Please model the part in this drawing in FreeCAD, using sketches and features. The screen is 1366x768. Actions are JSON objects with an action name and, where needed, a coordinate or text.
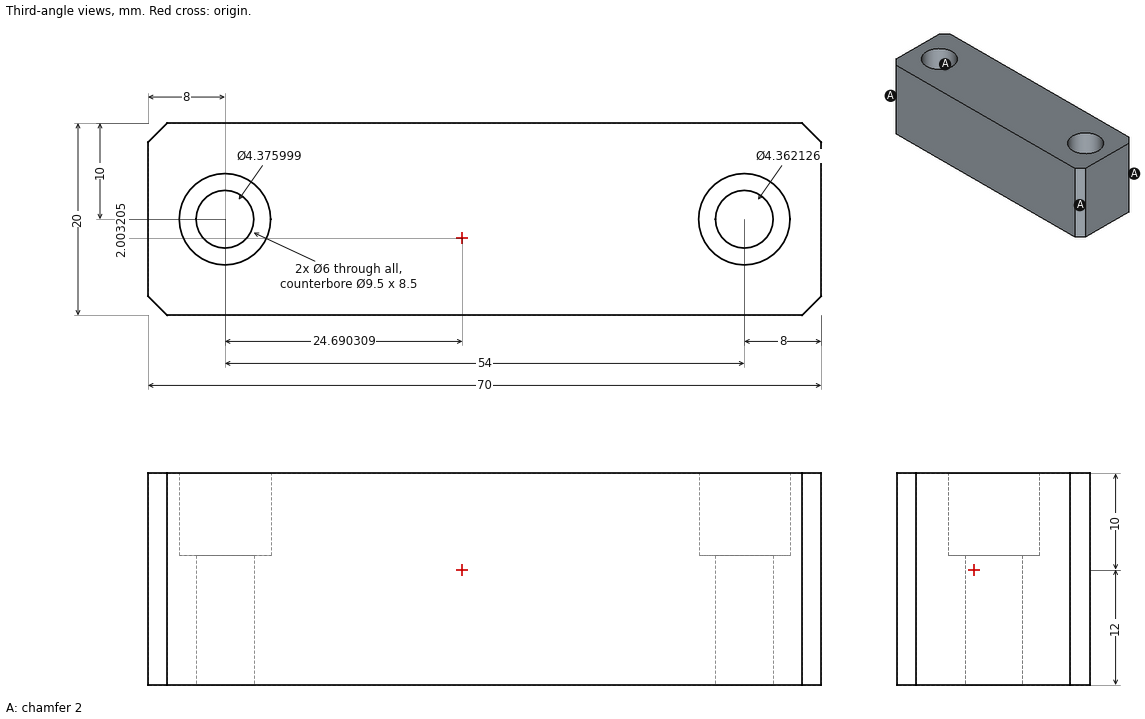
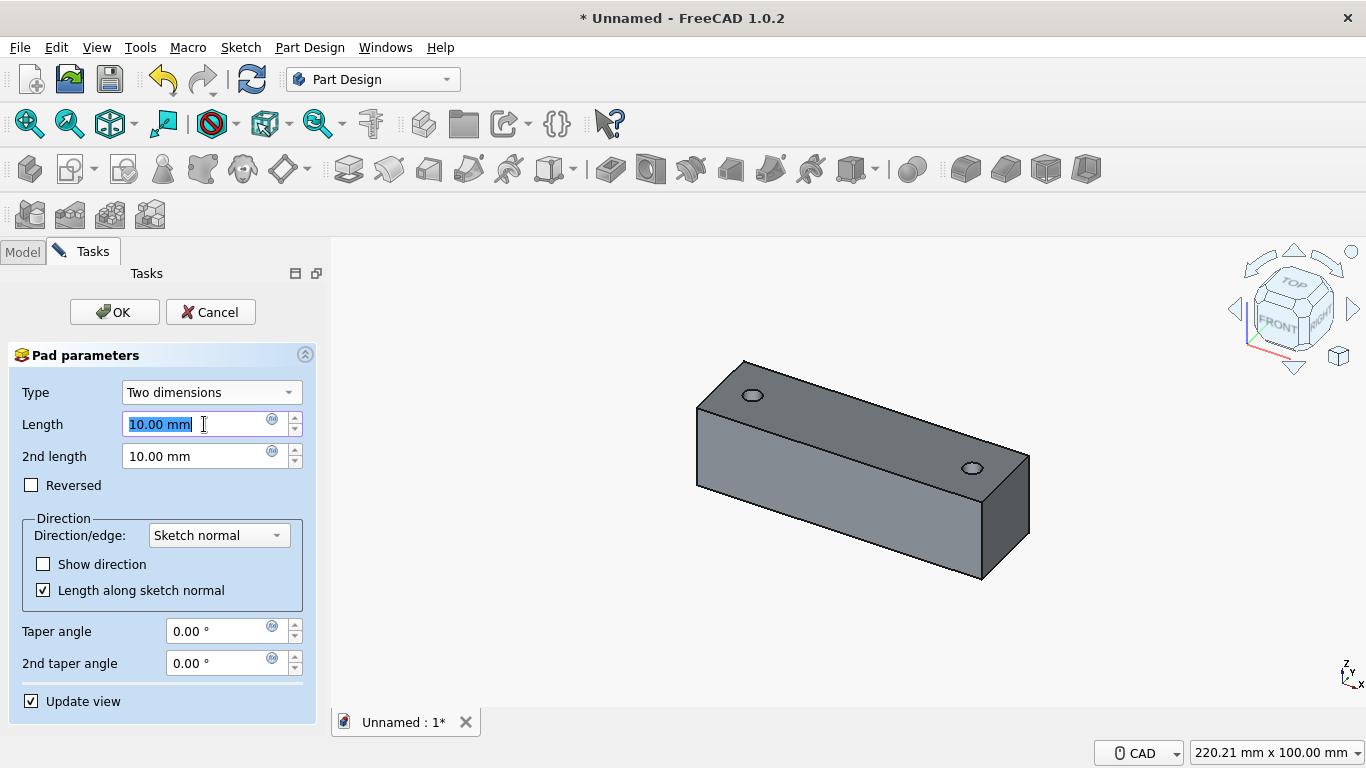
{"action": "type", "text": "10"}
{"action": "key", "text": "Tab"}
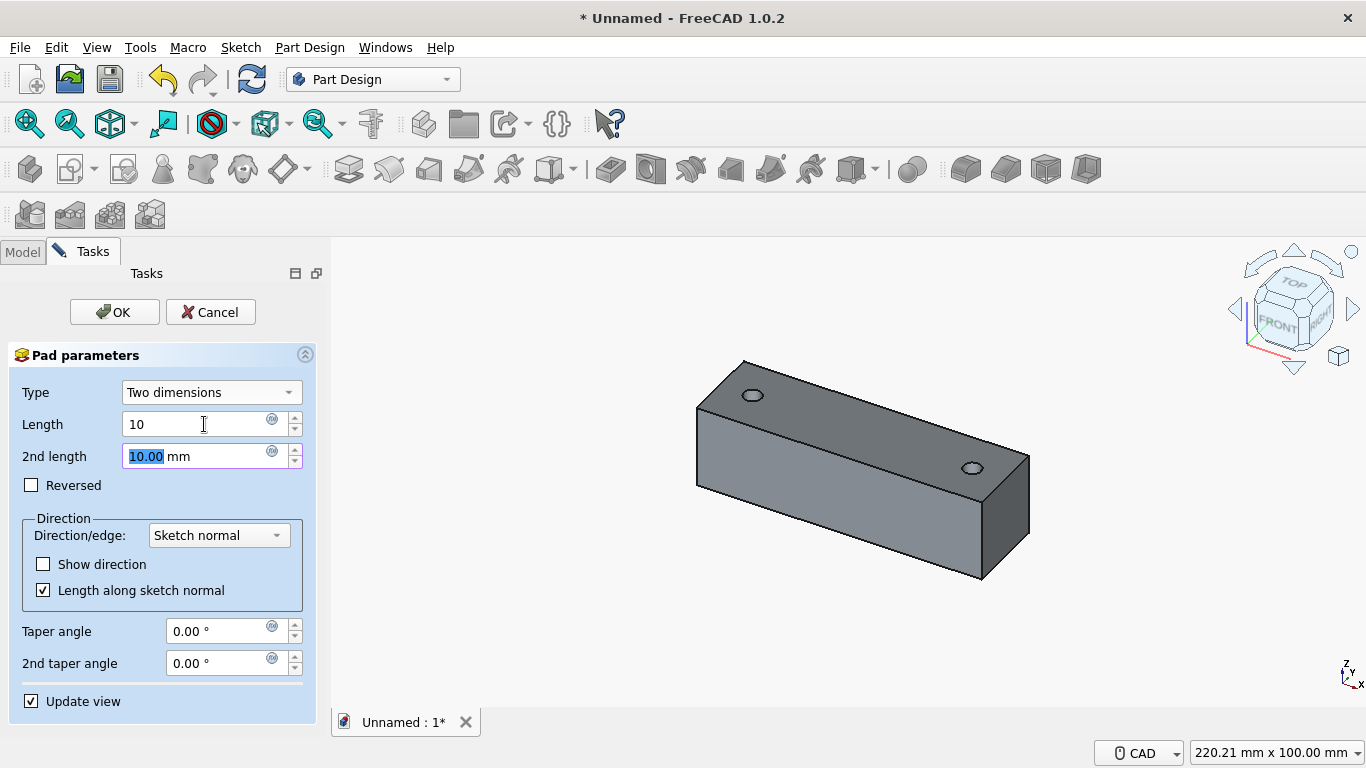
{"action": "type", "text": "12"}
{"action": "key", "text": "Tab"}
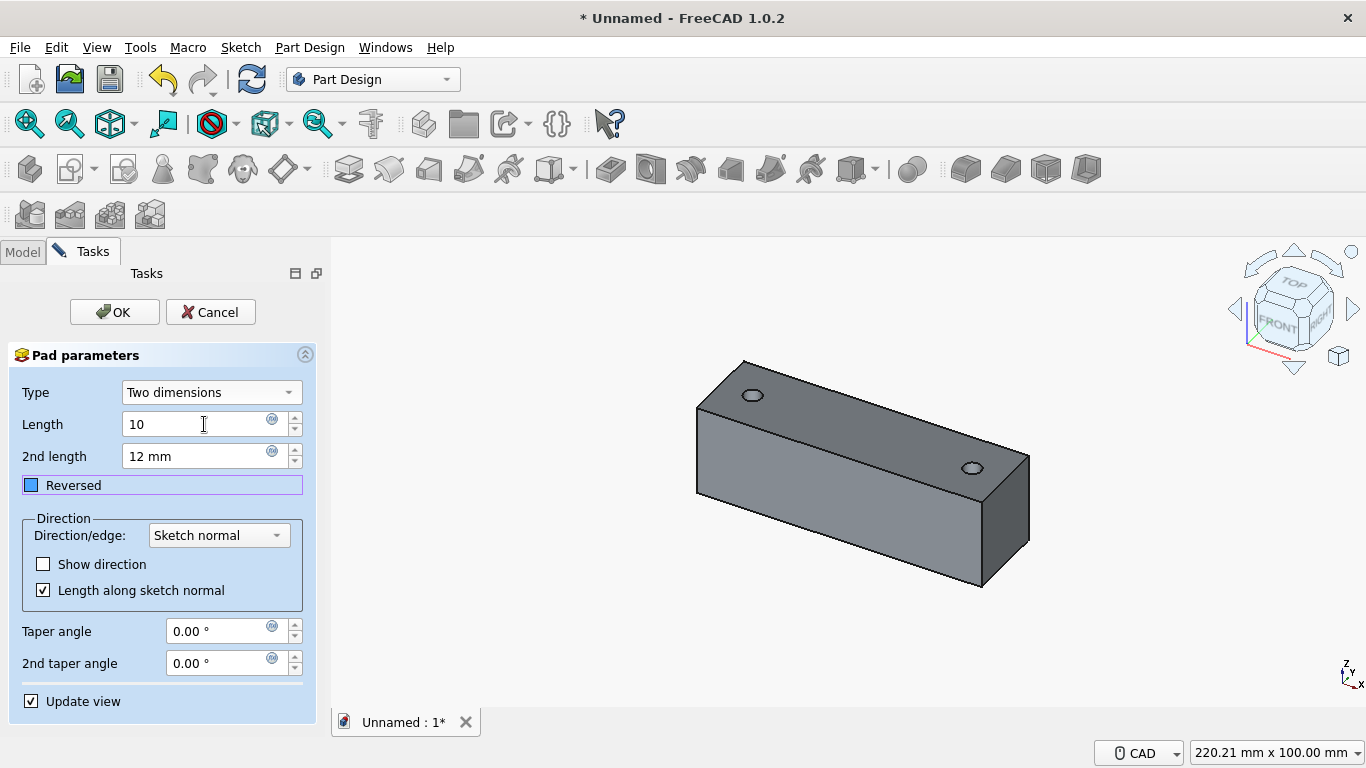
{"action": "left_click", "coordinate": [115, 312]}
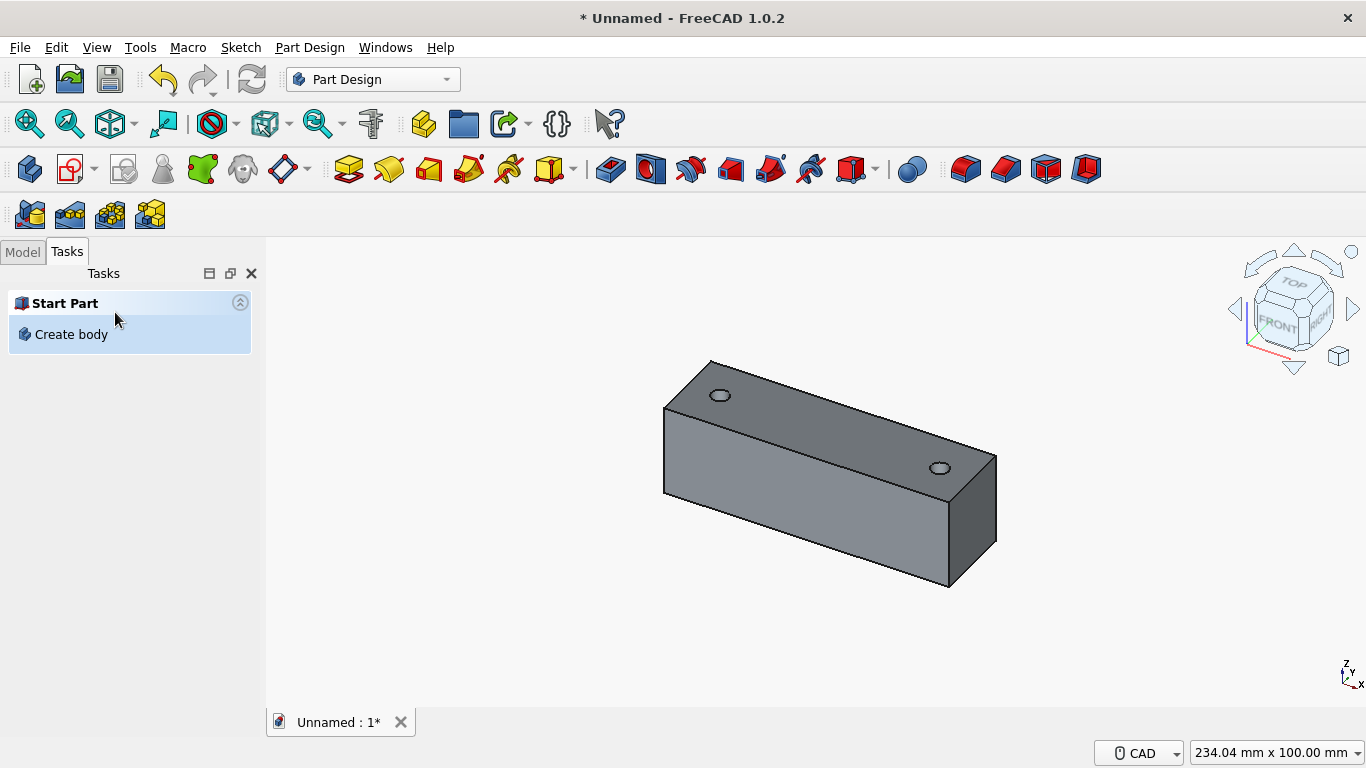
{"action": "left_click", "coordinate": [871, 444]}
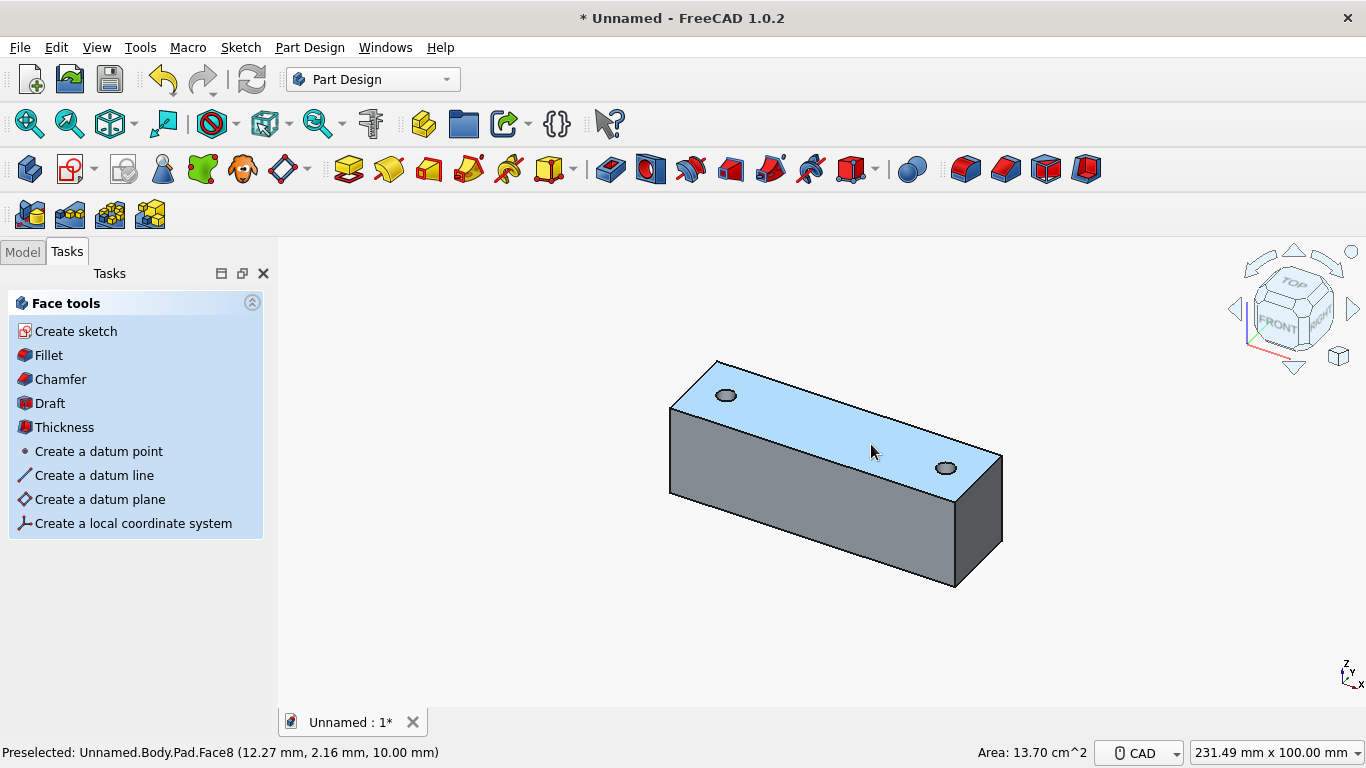
{"action": "left_click", "coordinate": [70, 170]}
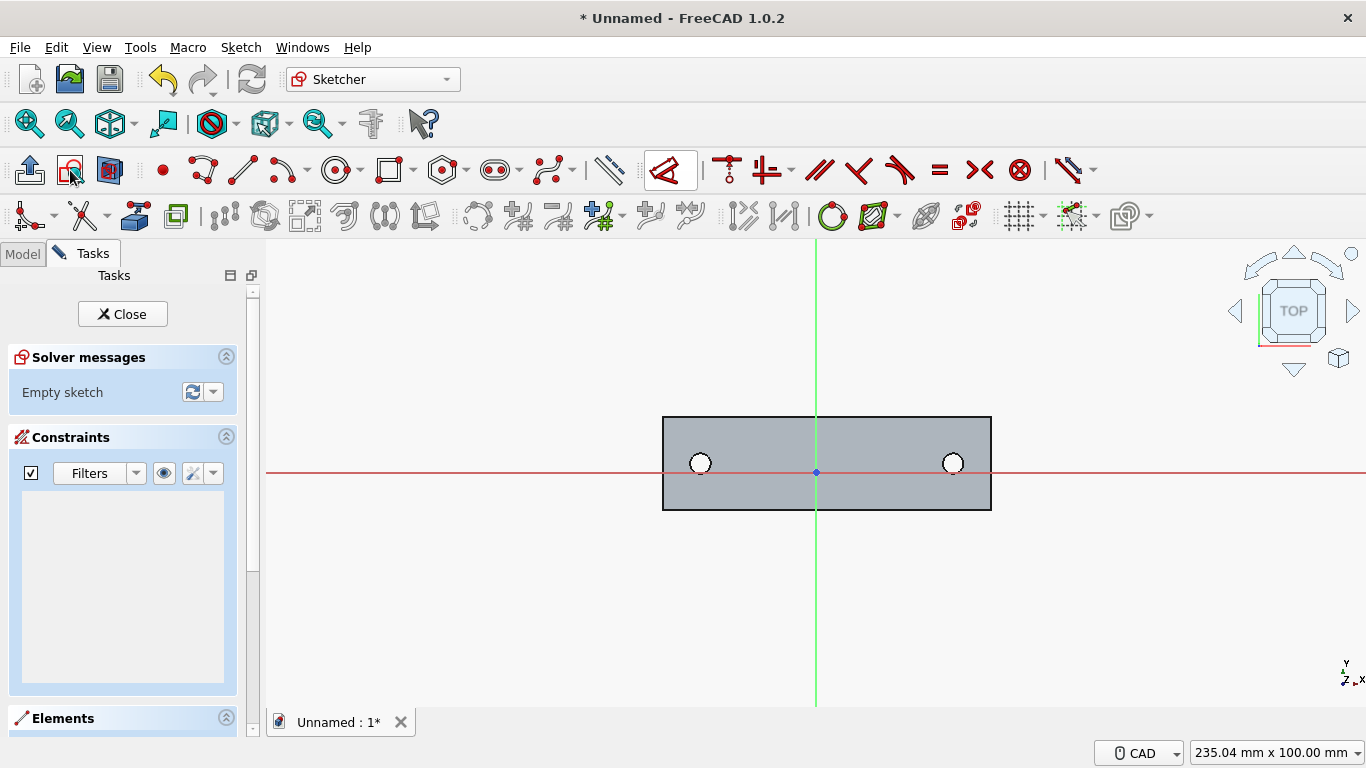
{"action": "scroll", "coordinate": [892, 456], "scroll_direction": "up", "scroll_amount": 4}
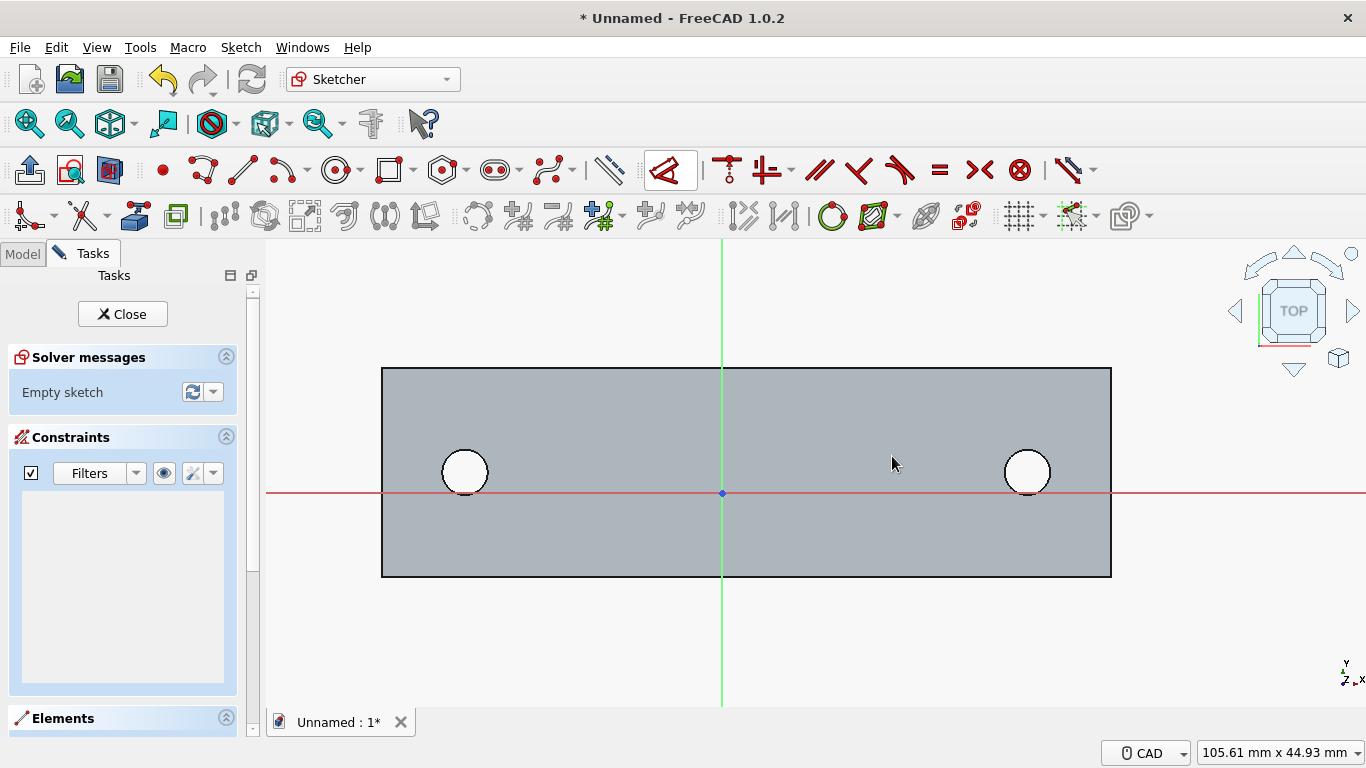
{"action": "left_click", "coordinate": [336, 170]}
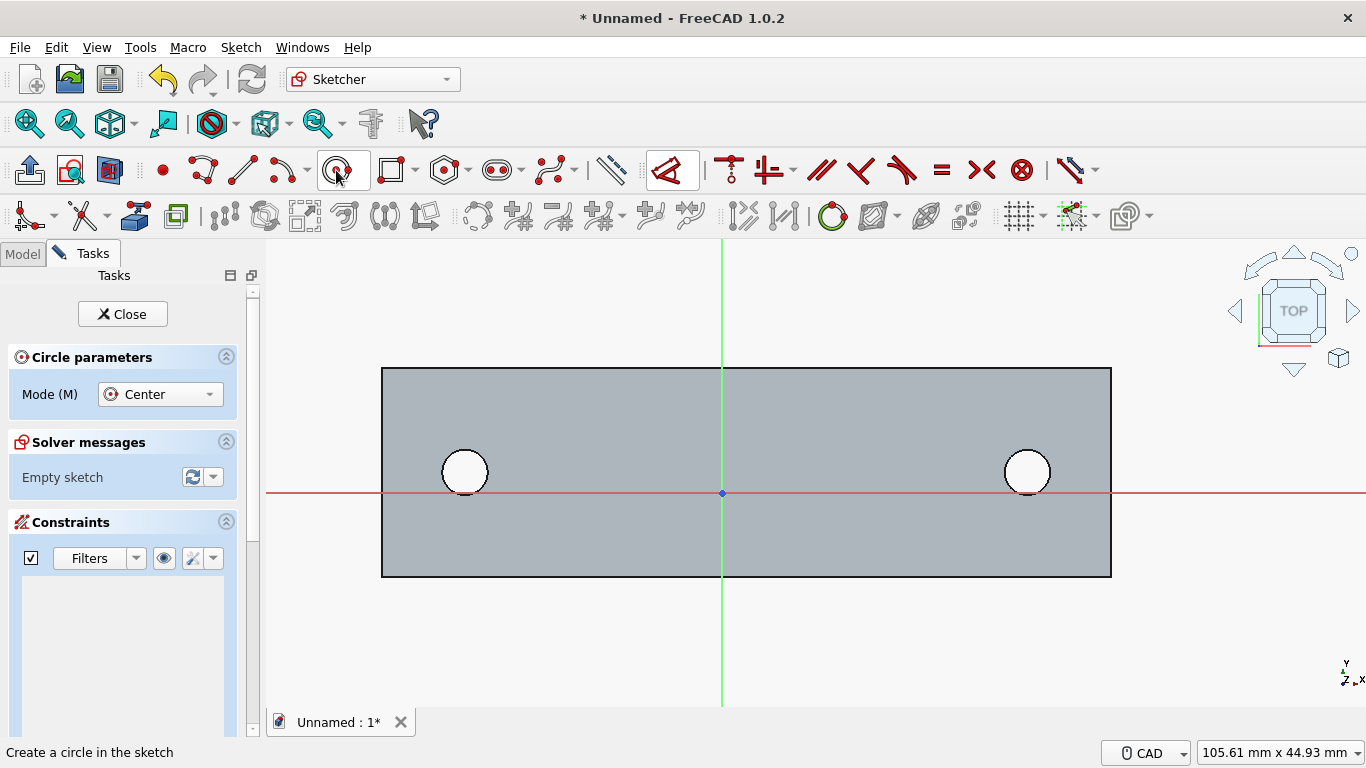
{"action": "left_click", "coordinate": [465, 472]}
{"action": "left_click", "coordinate": [487, 450]}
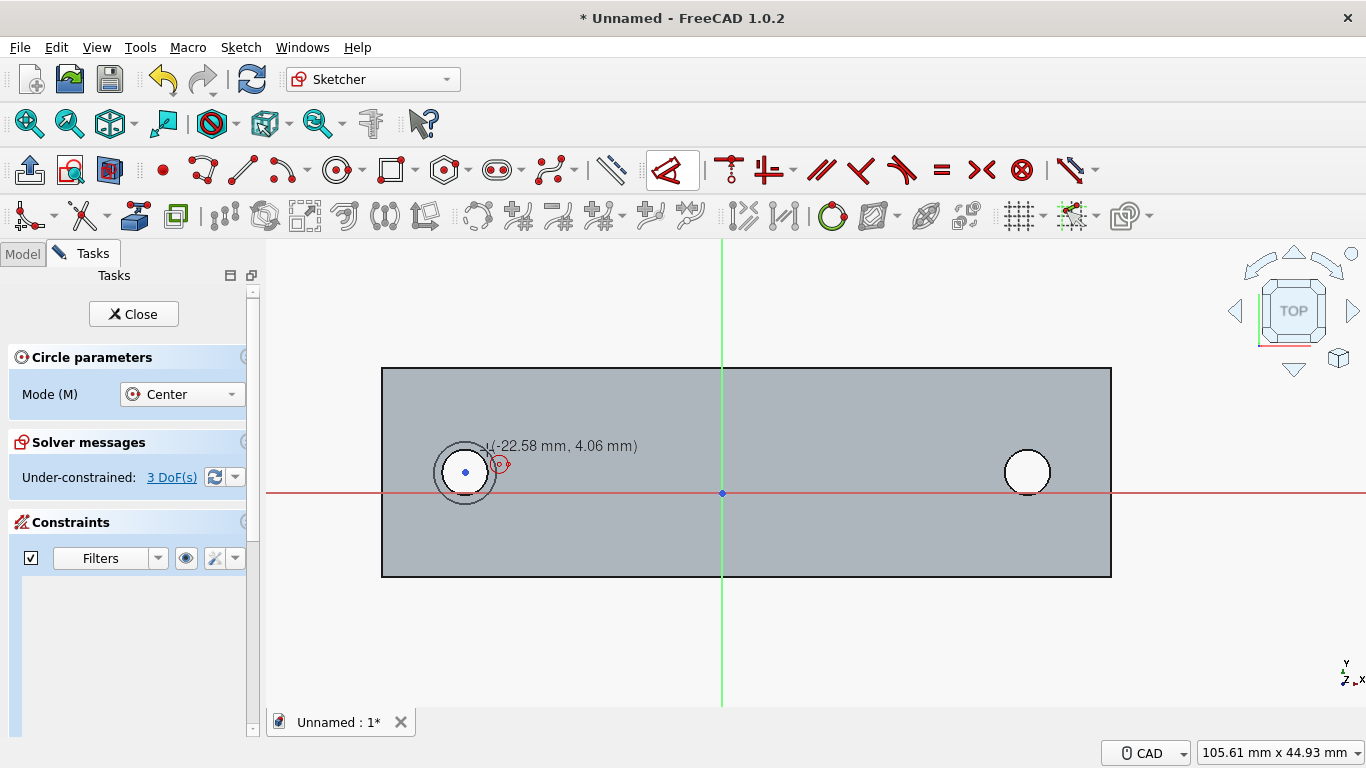
{"action": "left_click", "coordinate": [1027, 472]}
{"action": "left_click", "coordinate": [1050, 450]}
{"action": "key", "text": "Escape"}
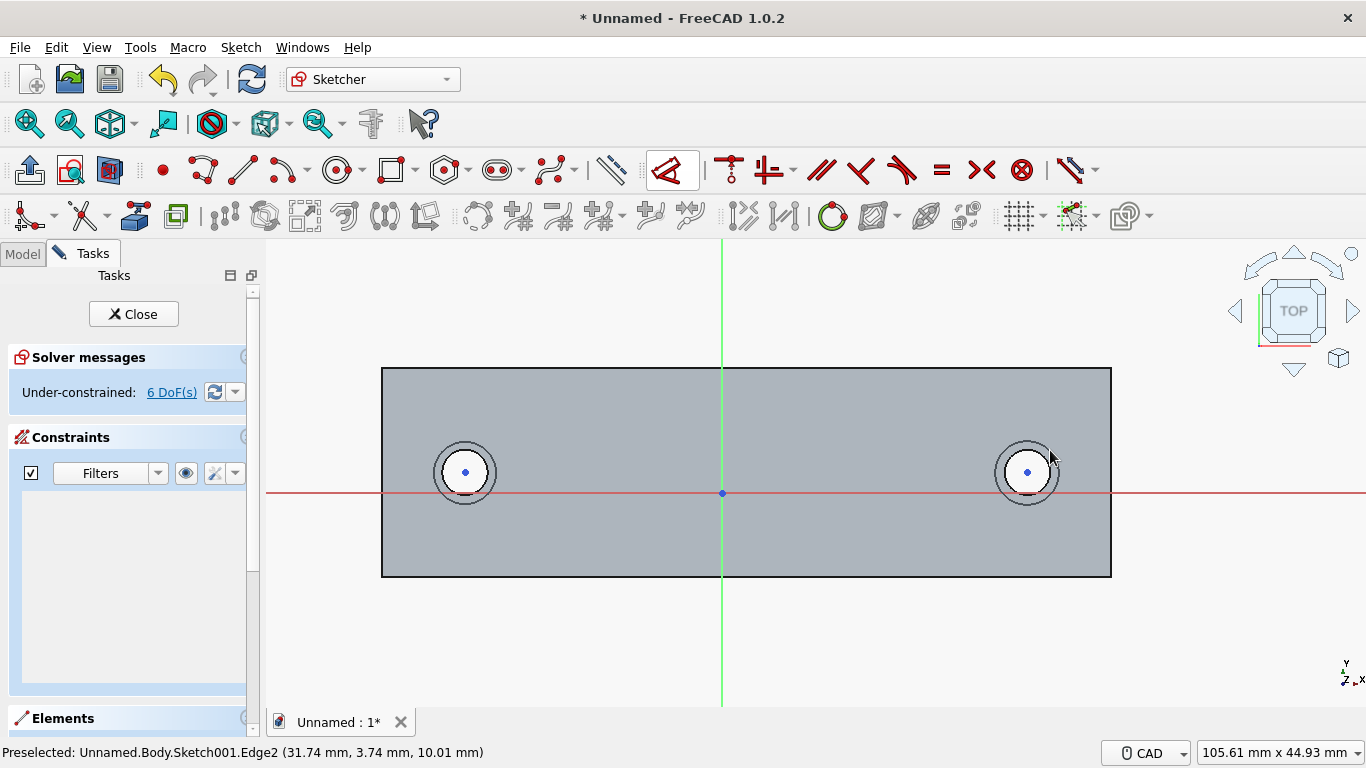
{"action": "left_click", "coordinate": [487, 451]}